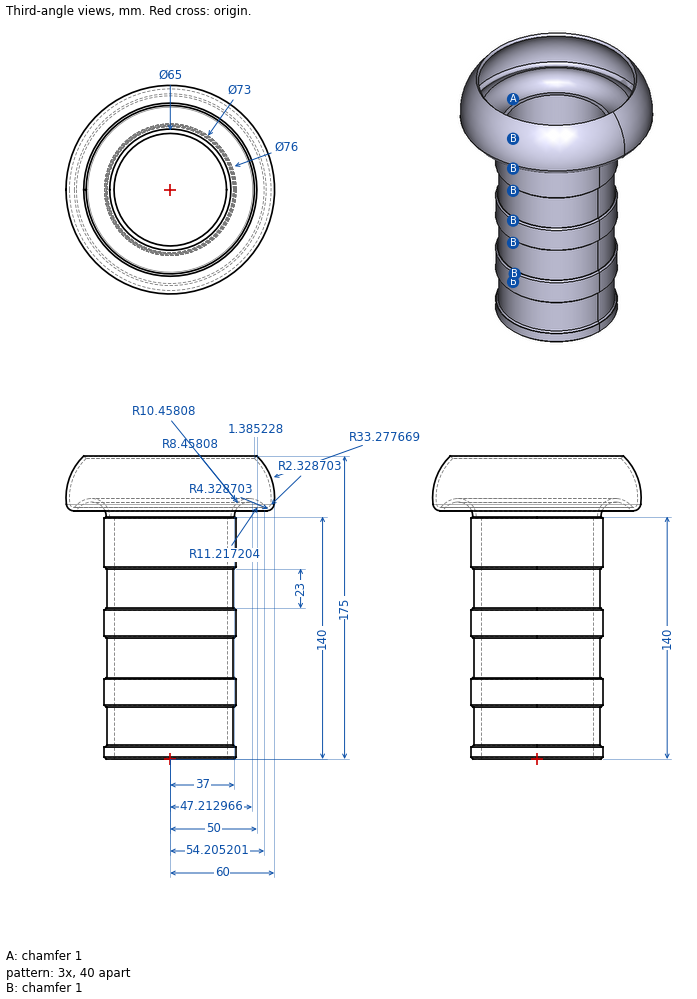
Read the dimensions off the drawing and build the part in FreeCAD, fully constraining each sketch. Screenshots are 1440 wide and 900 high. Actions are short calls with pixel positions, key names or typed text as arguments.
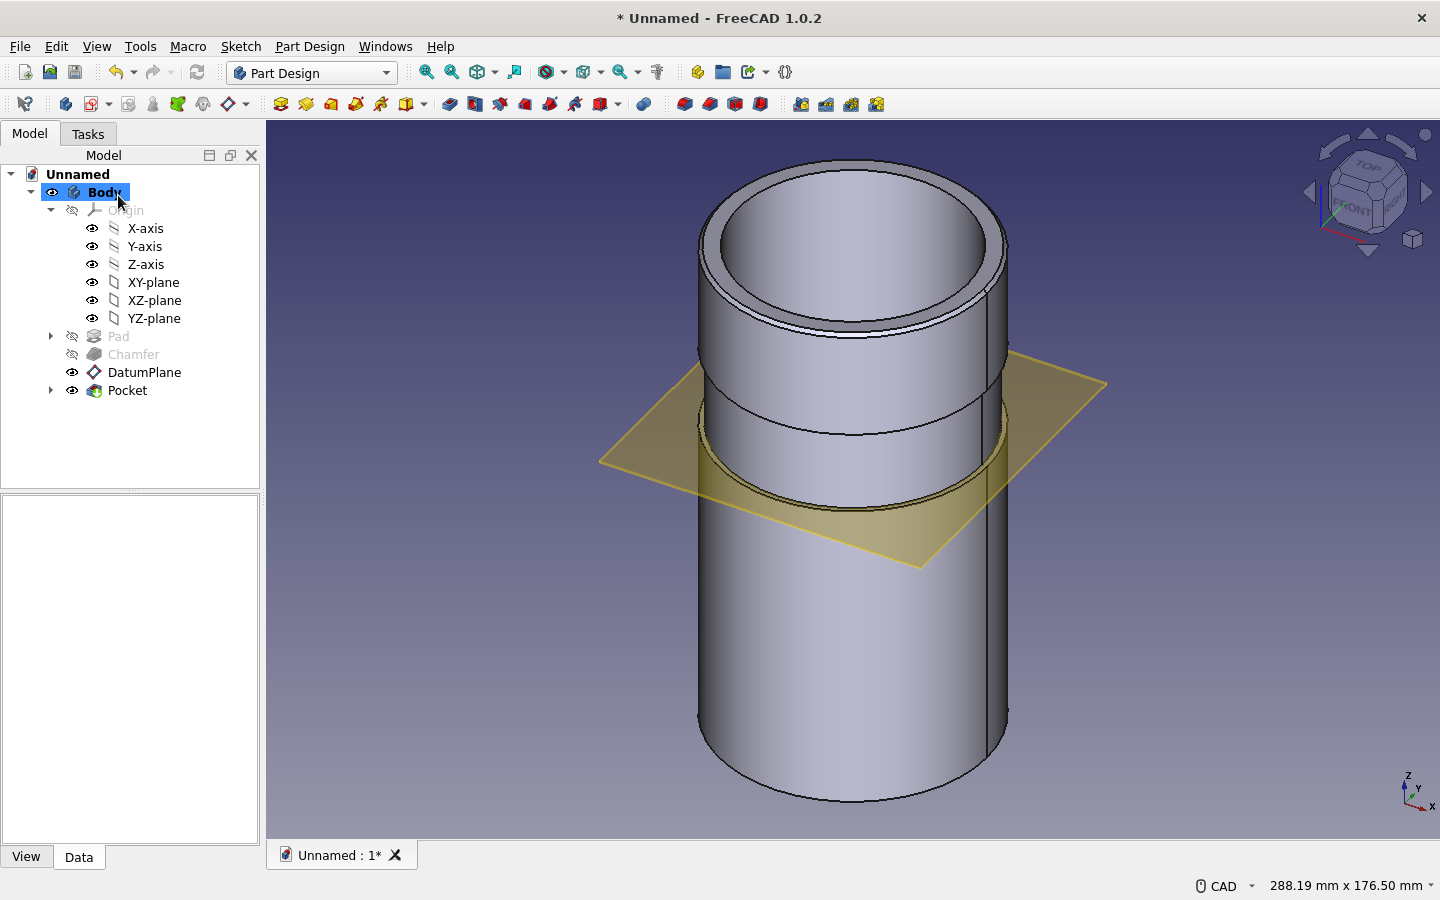
click(117, 372)
key(space)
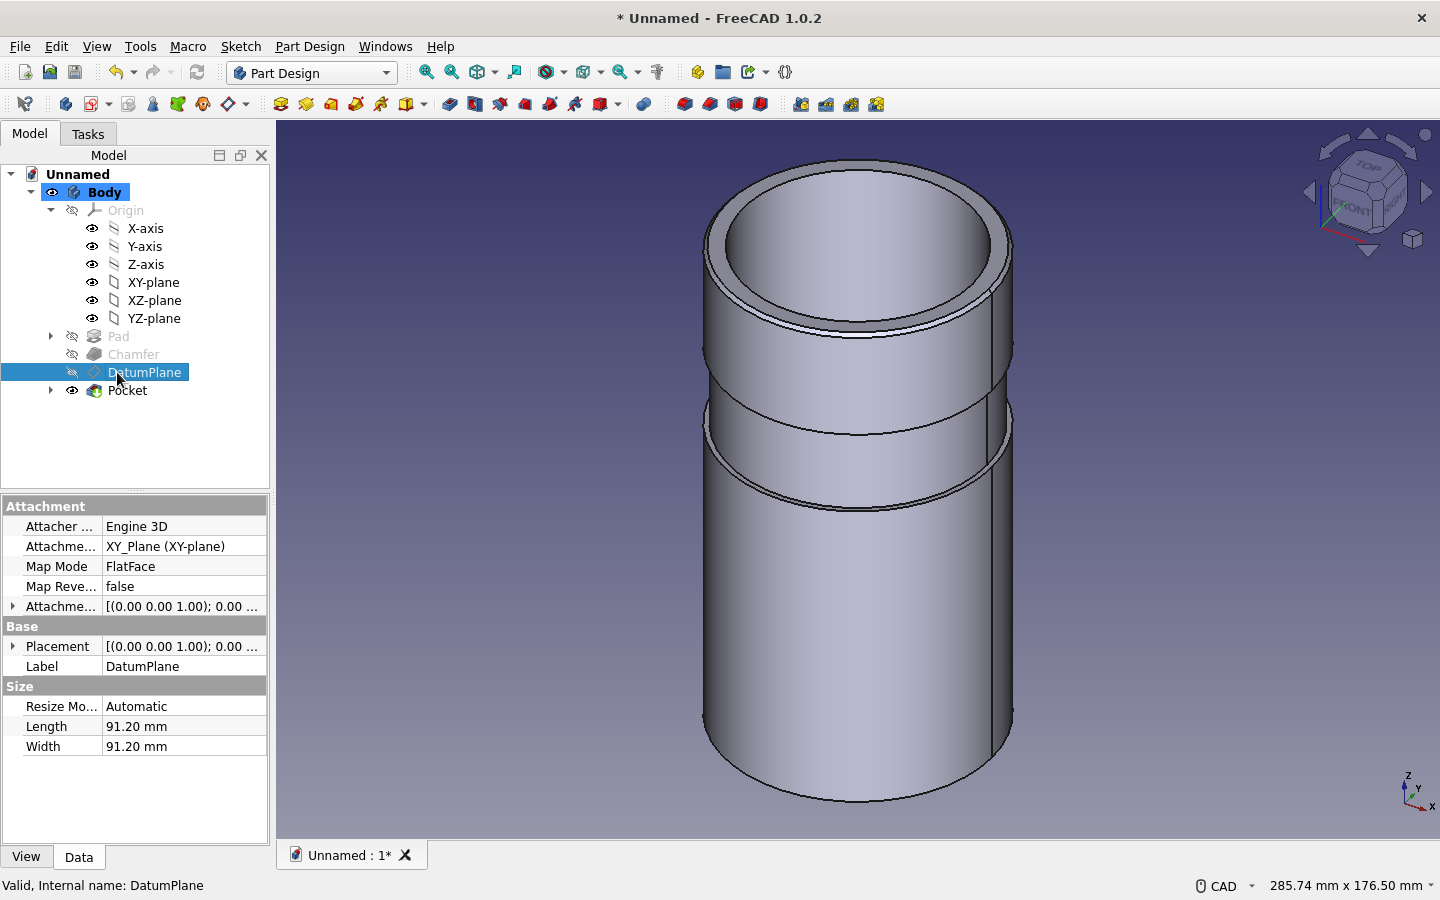
click(117, 390)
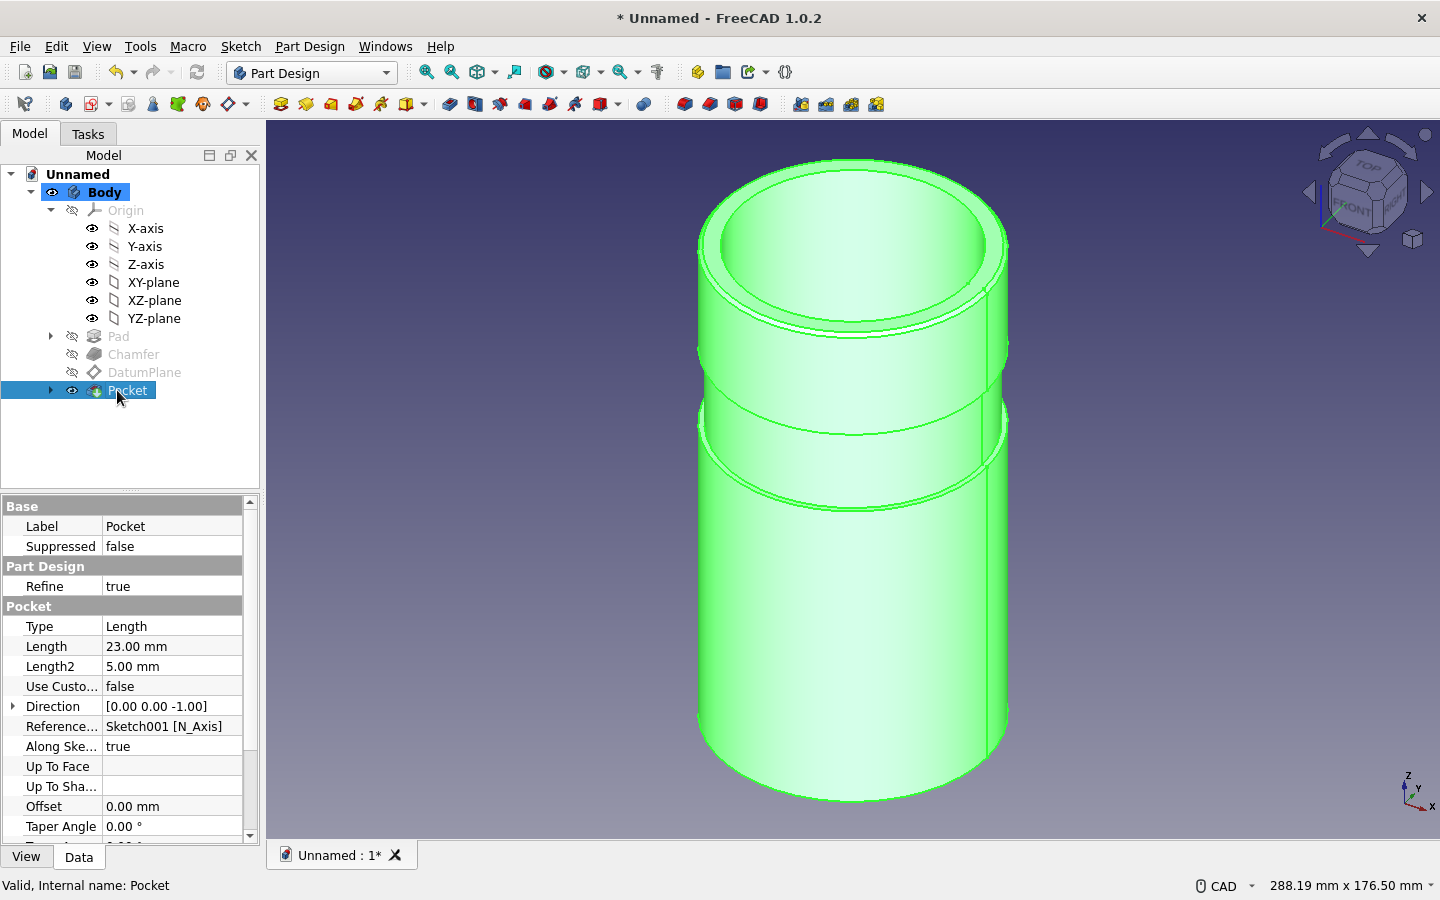
click(826, 104)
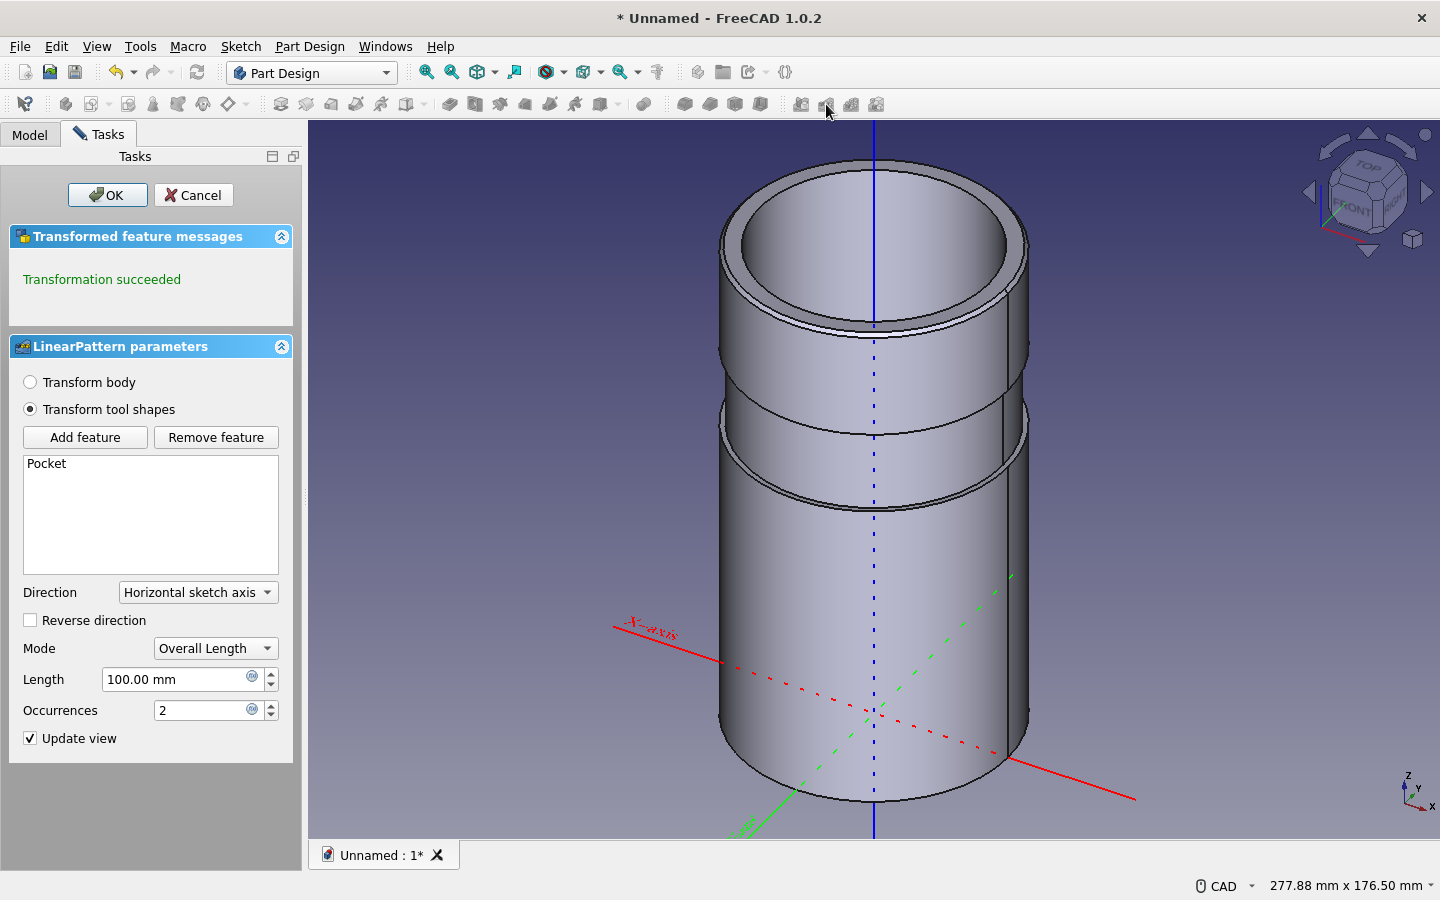
click(199, 592)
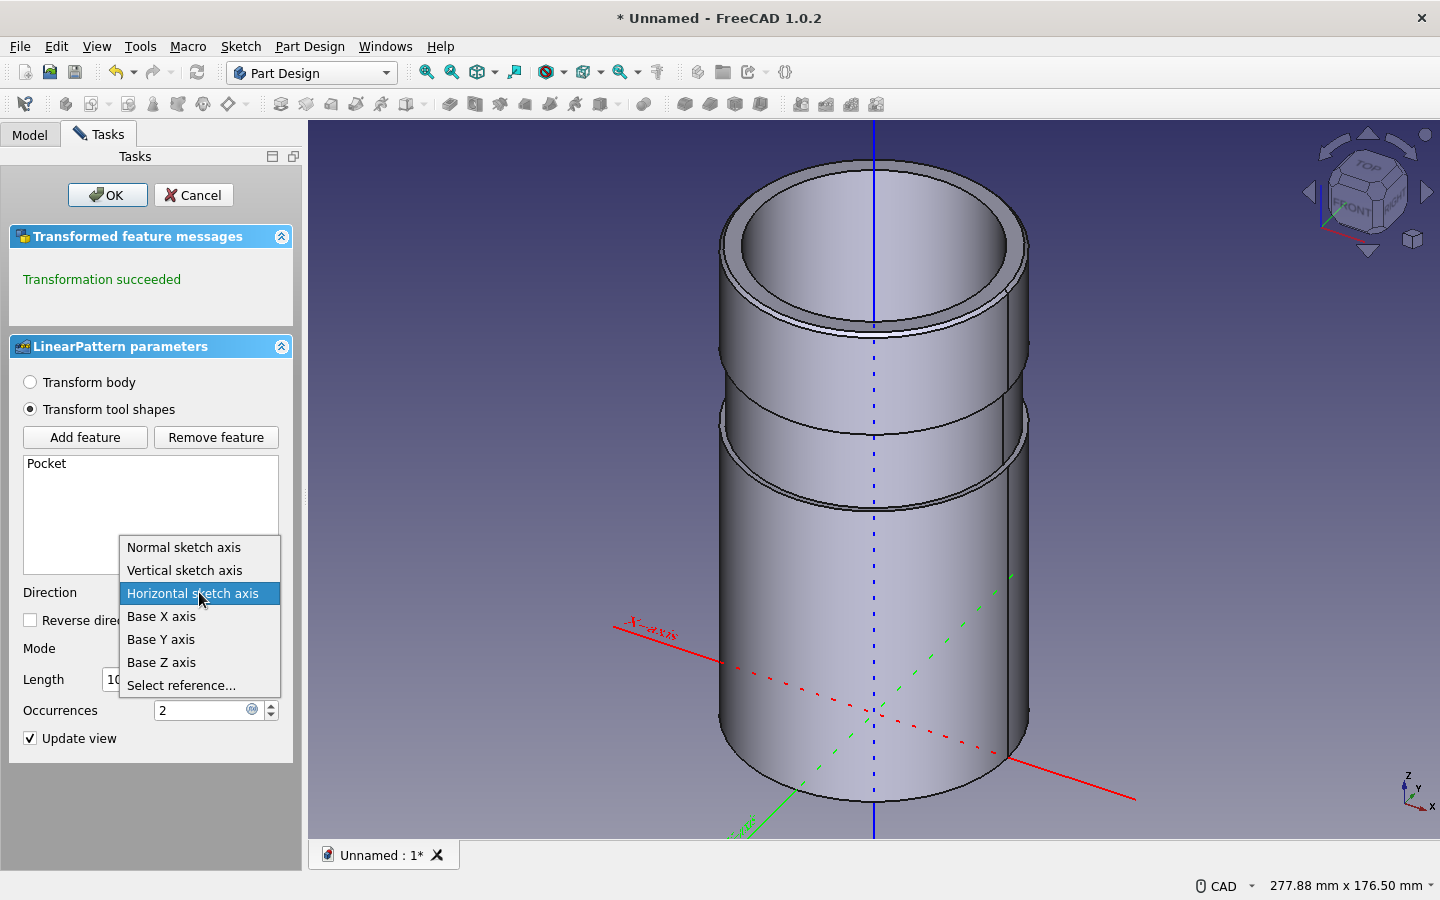
click(198, 662)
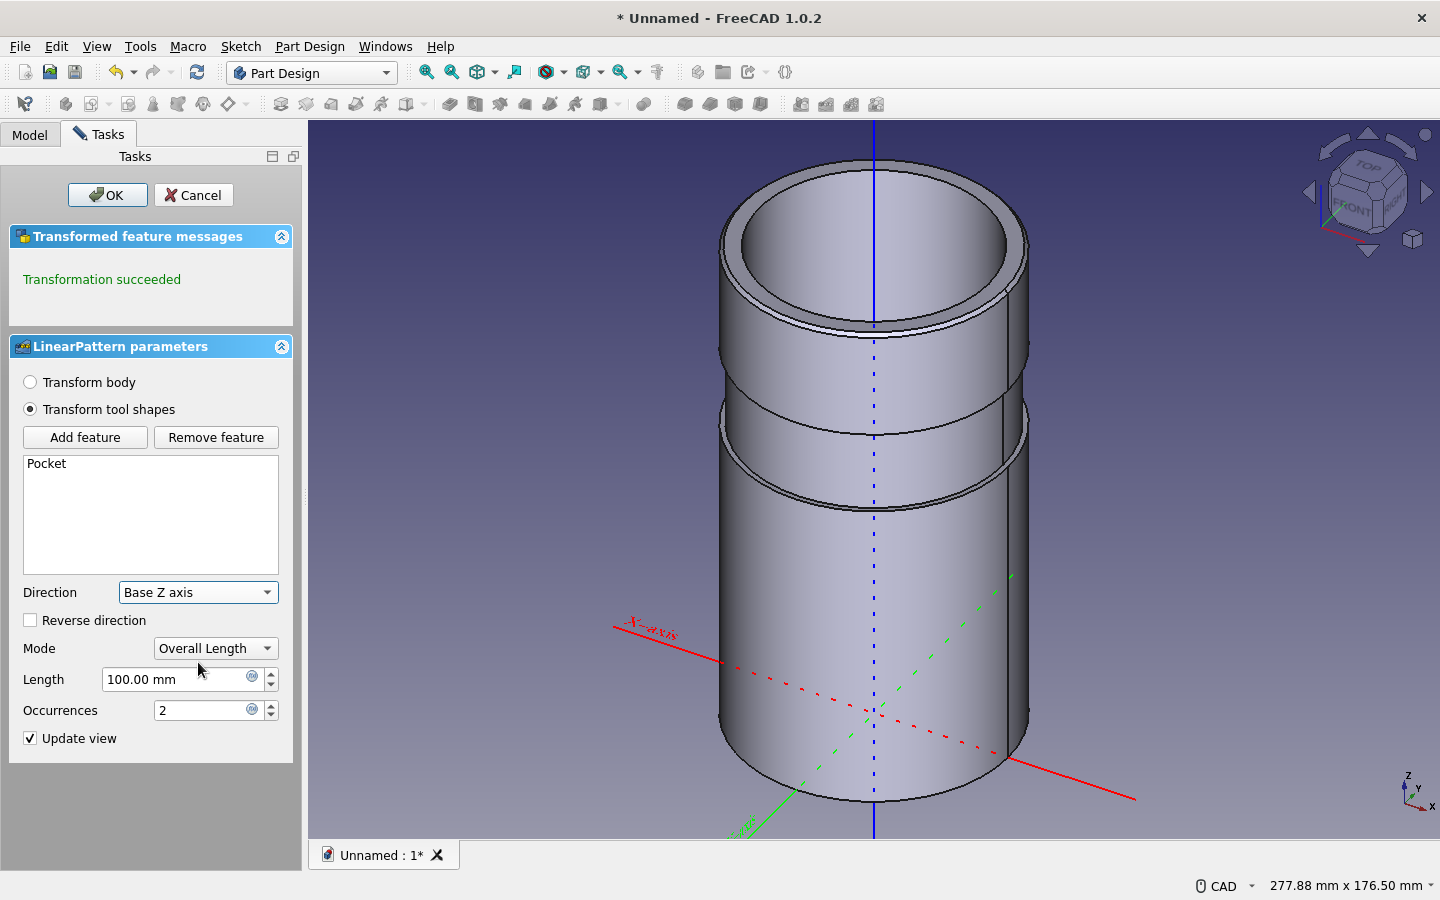
click(216, 648)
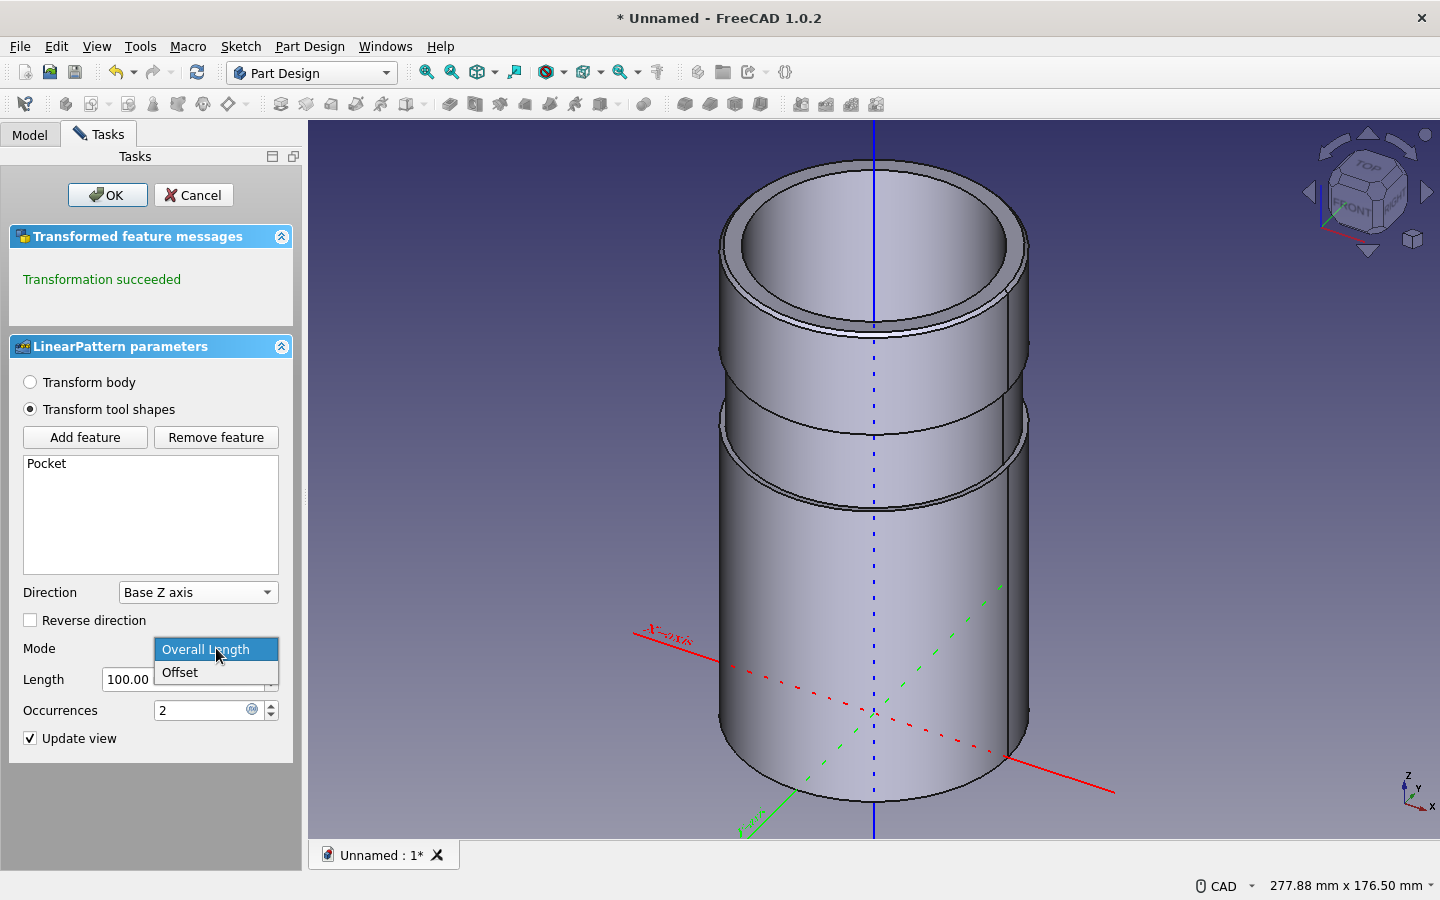
click(214, 672)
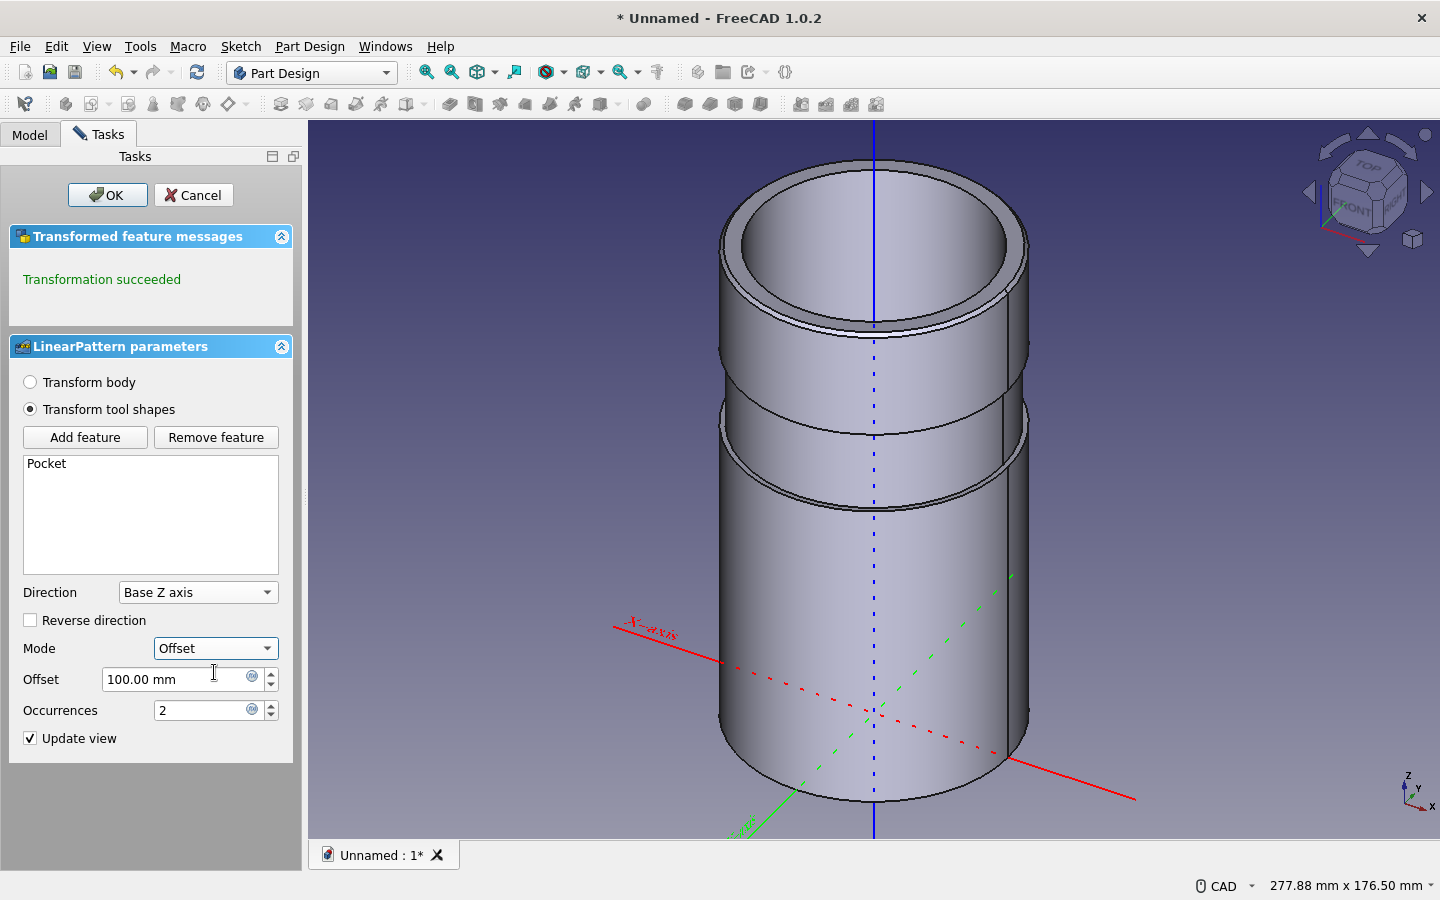
triple_click(184, 680)